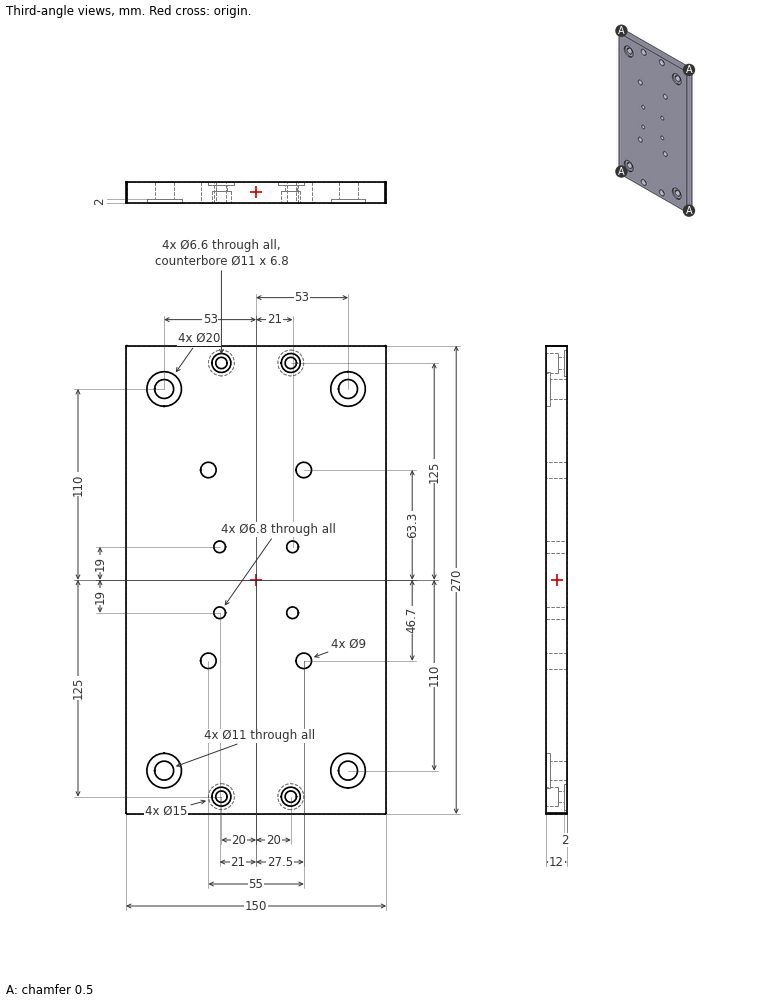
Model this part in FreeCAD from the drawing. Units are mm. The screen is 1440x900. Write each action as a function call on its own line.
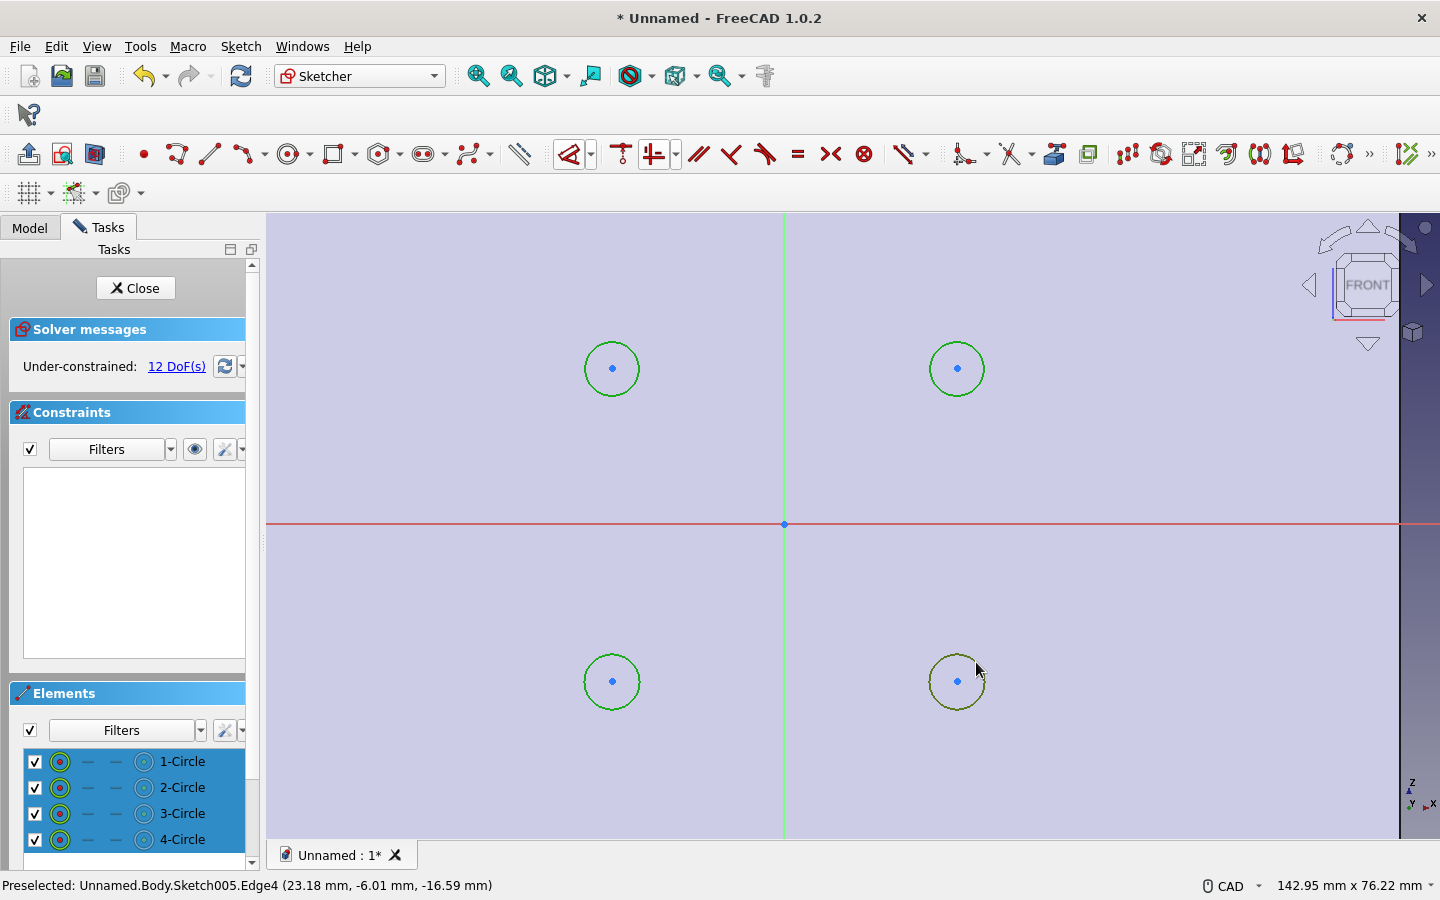
key(e)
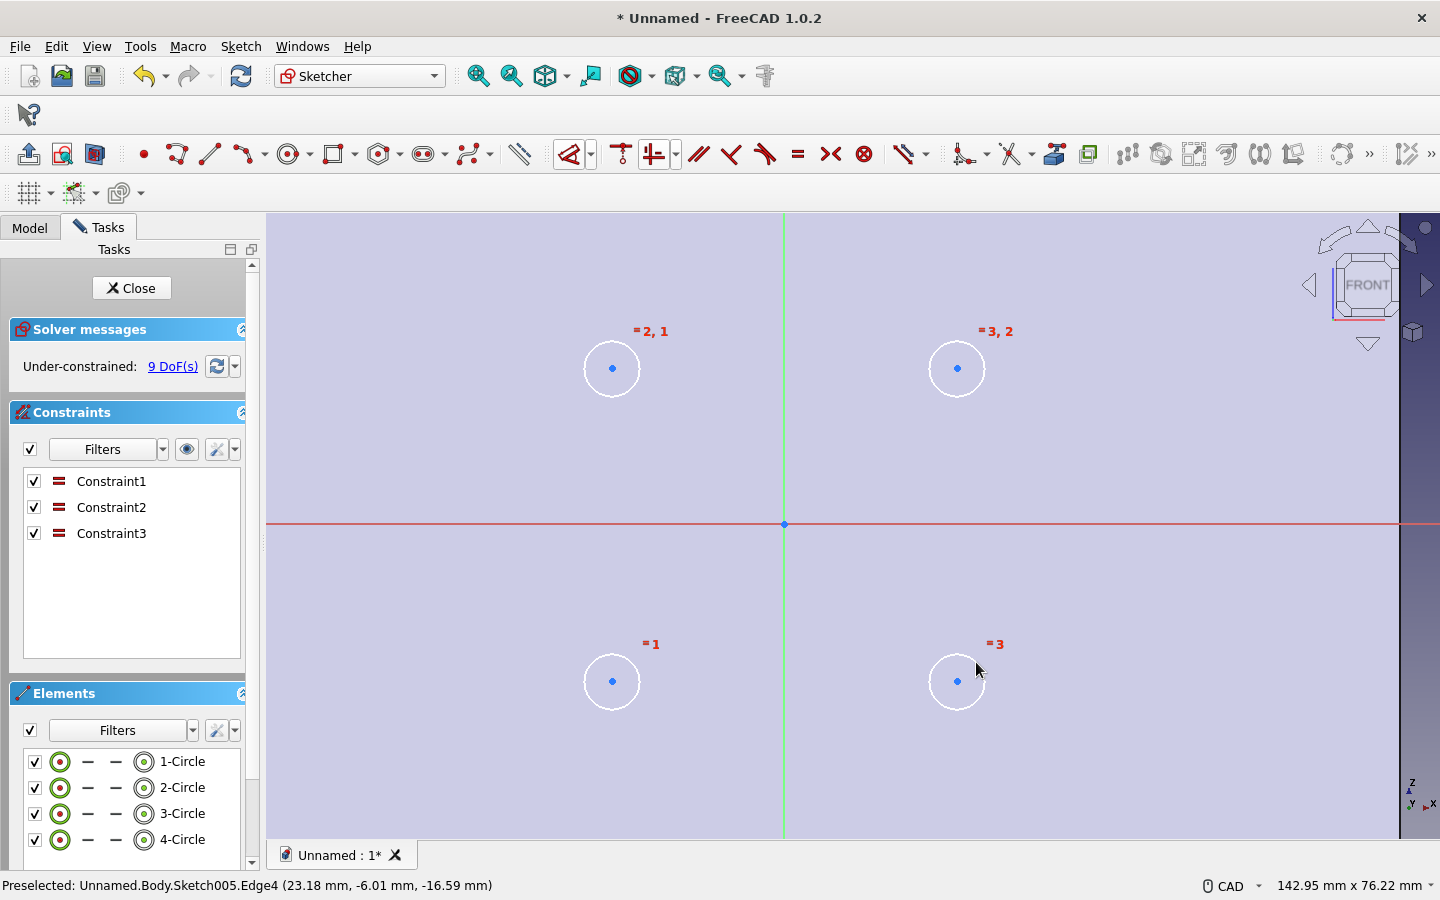
click(612, 682)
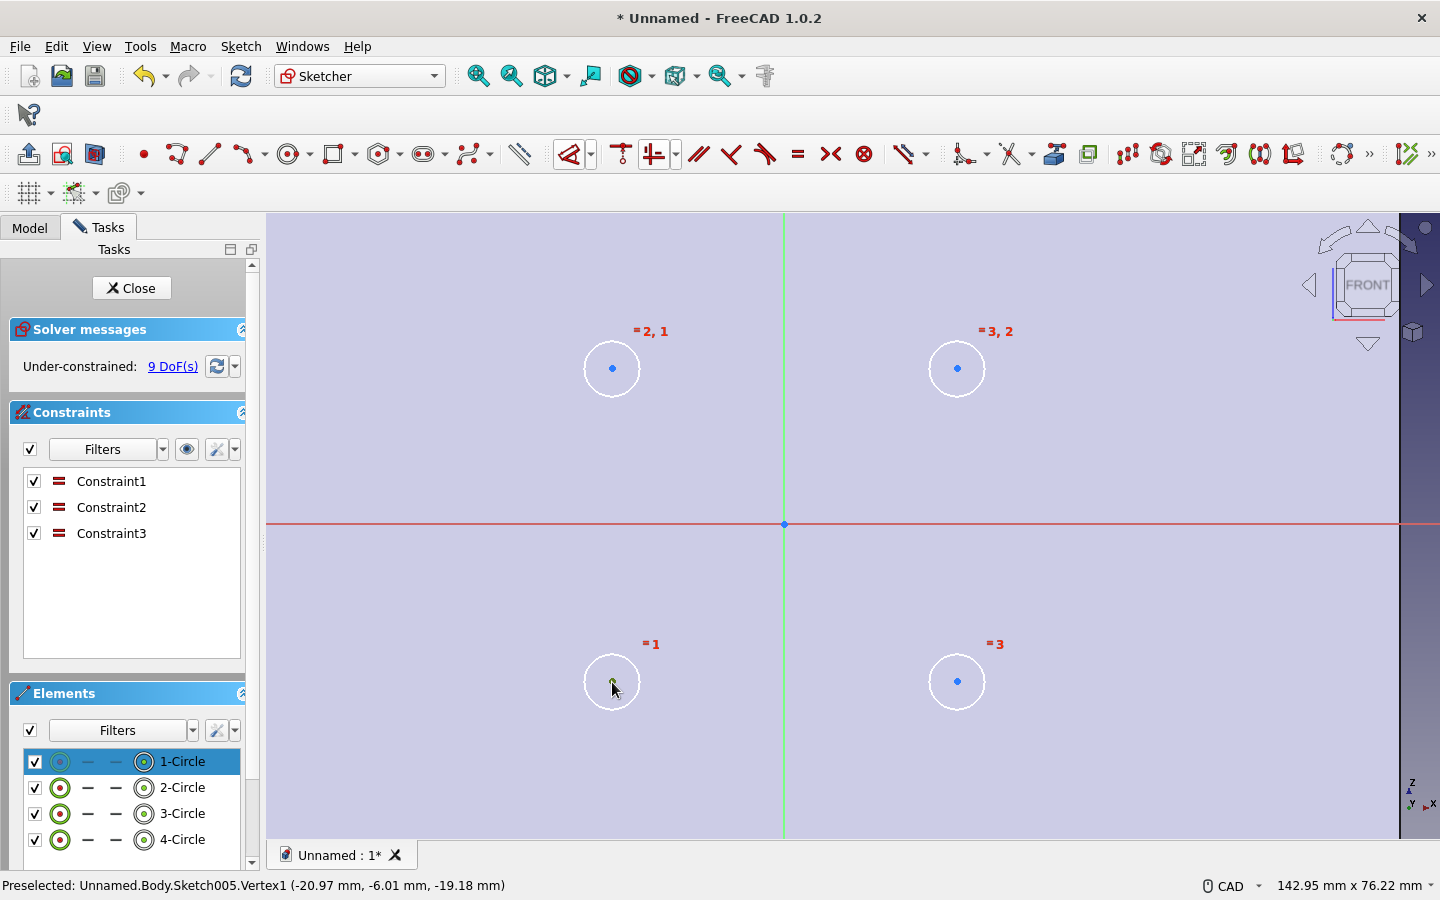
click(612, 369)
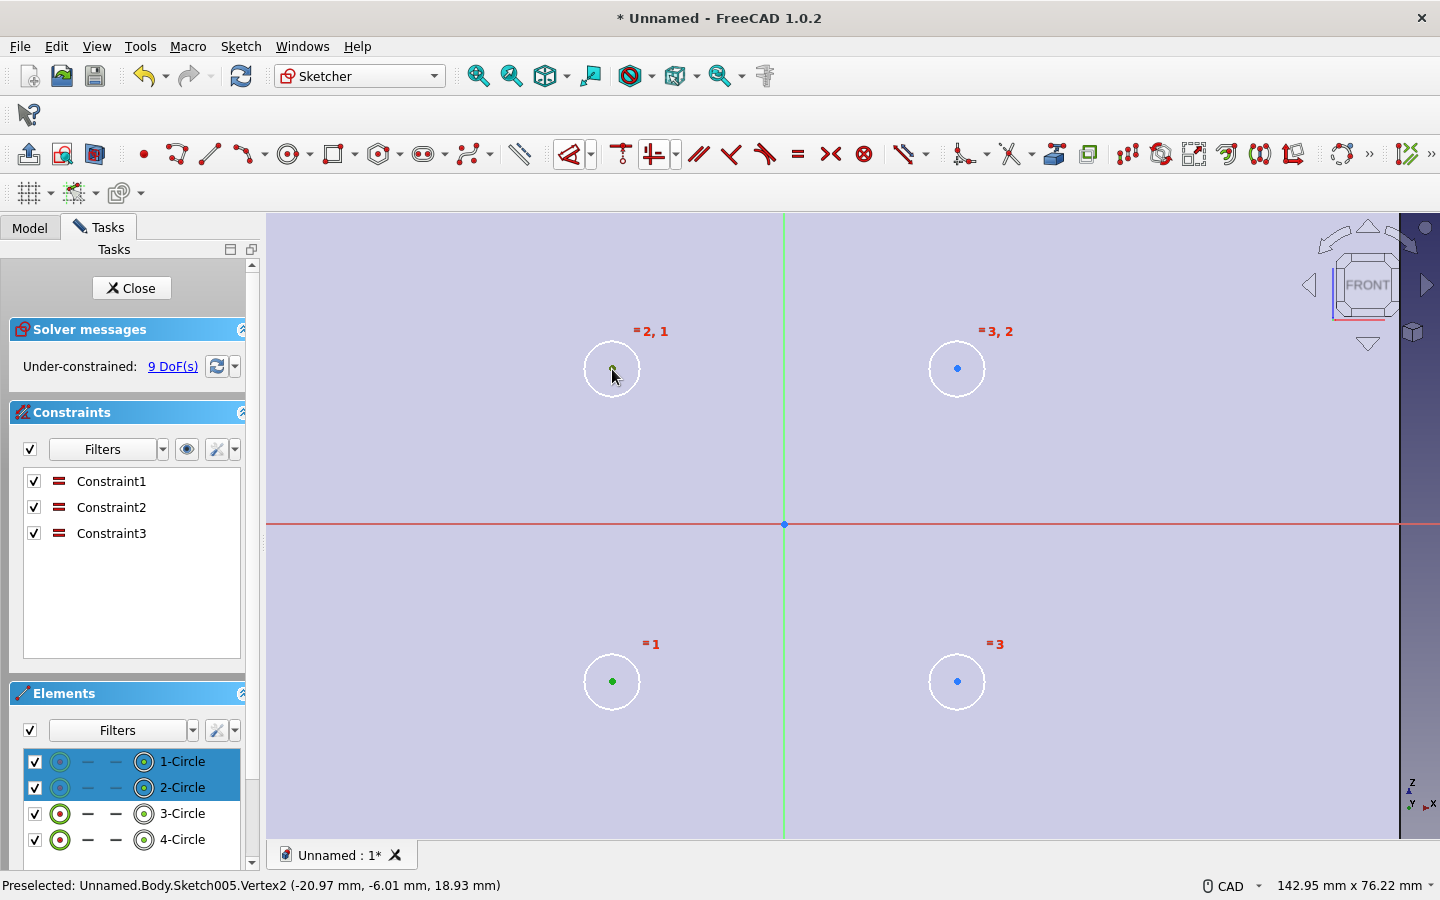
key(v)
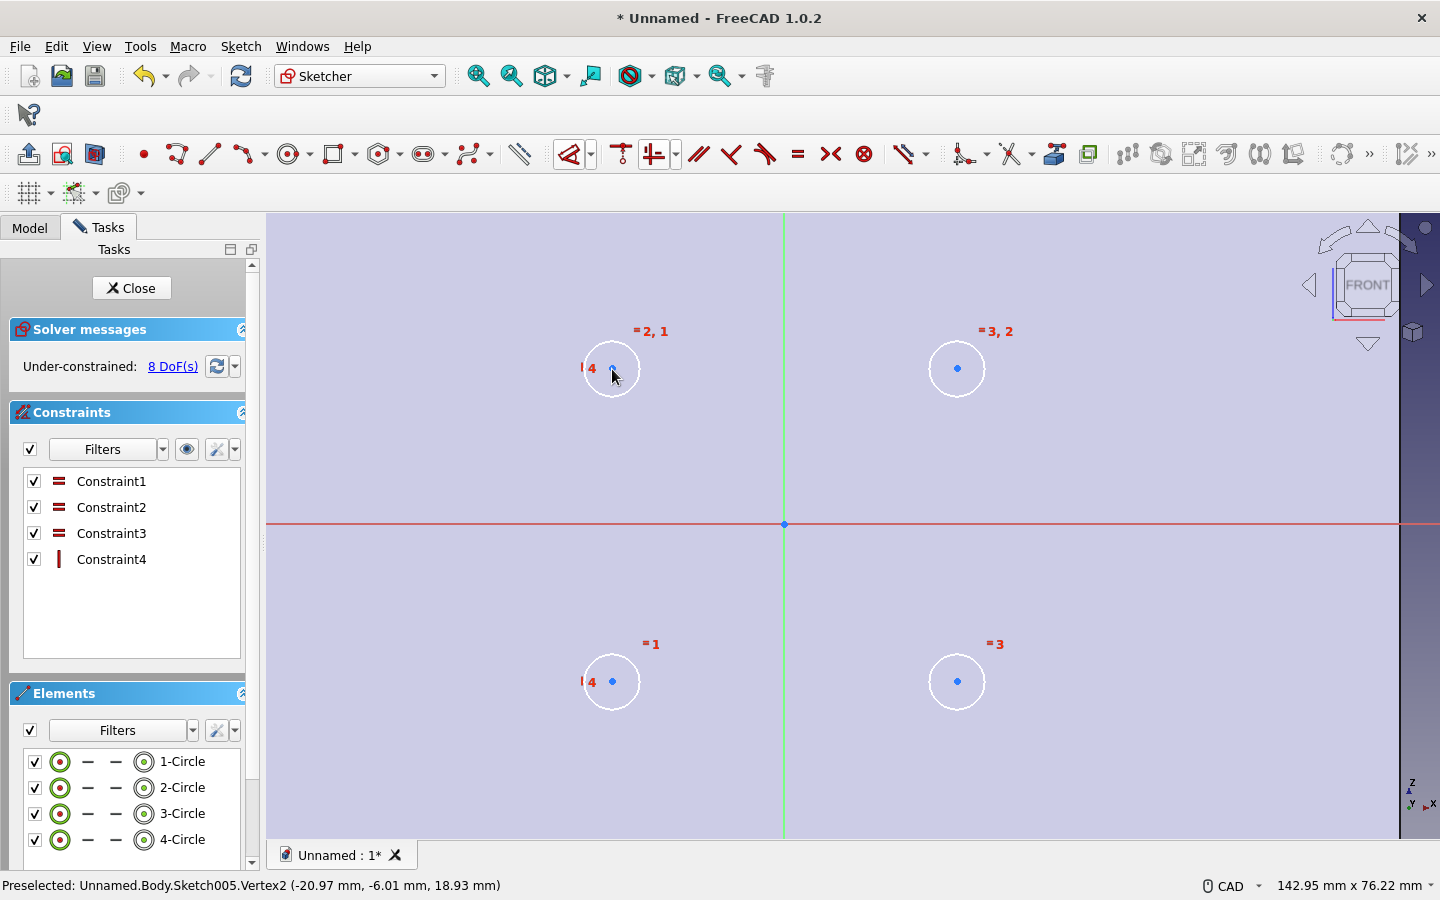
click(612, 369)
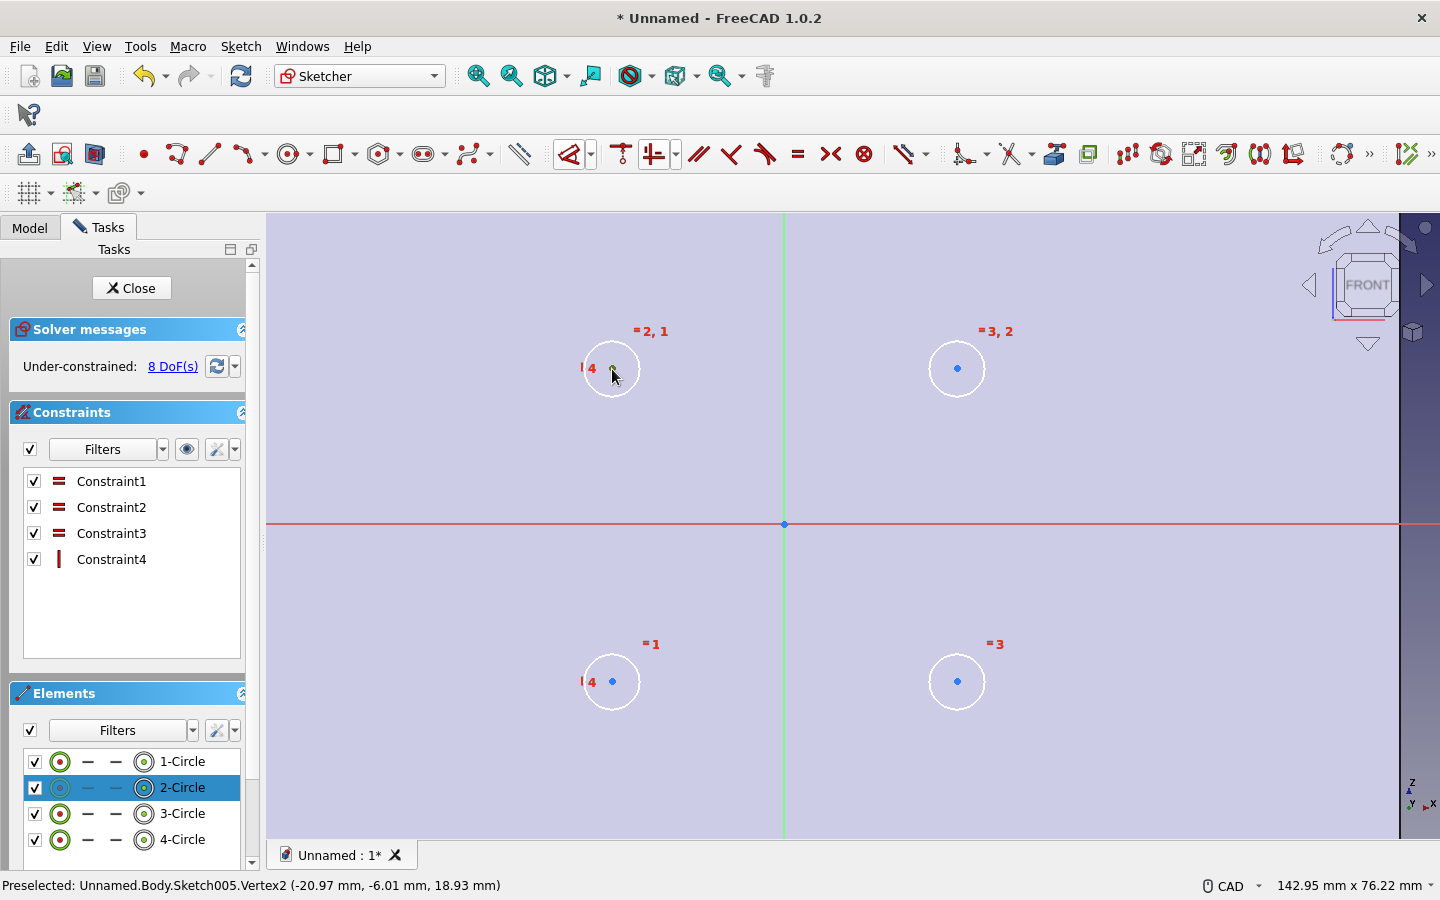
click(957, 369)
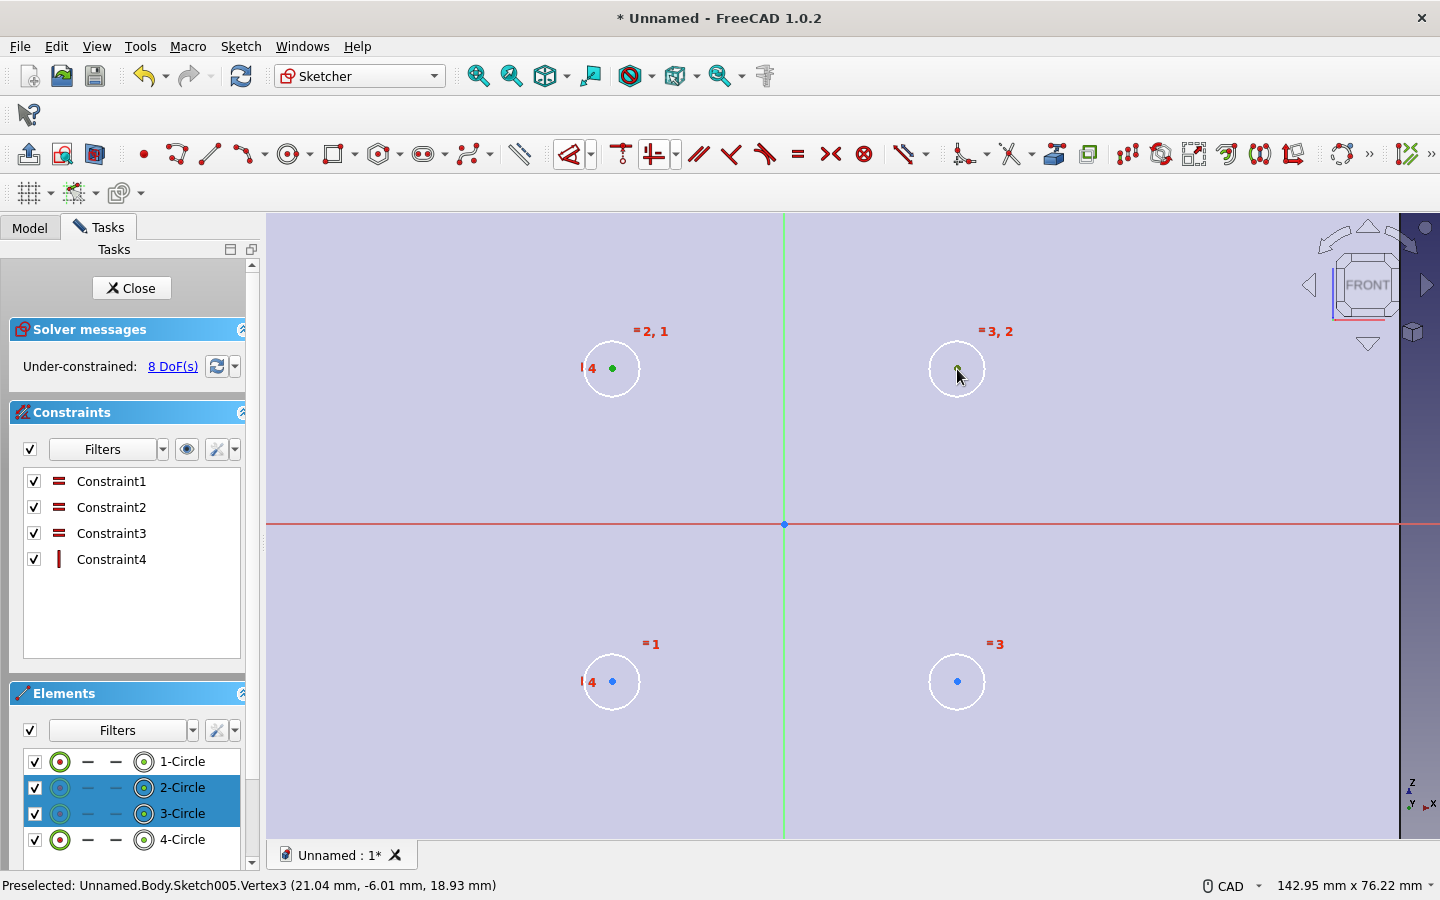
key(h)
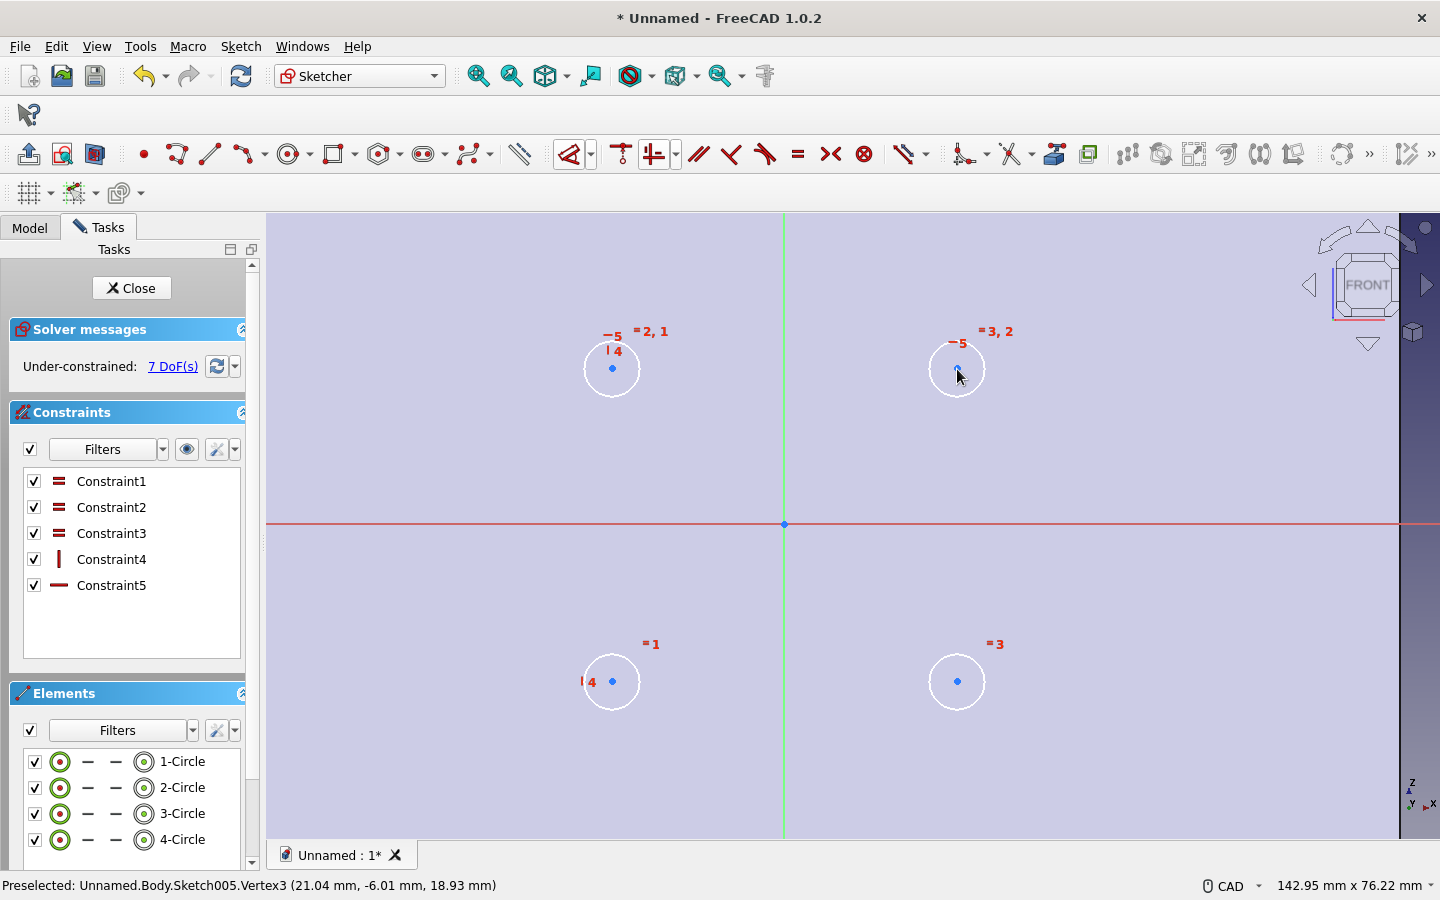
click(957, 369)